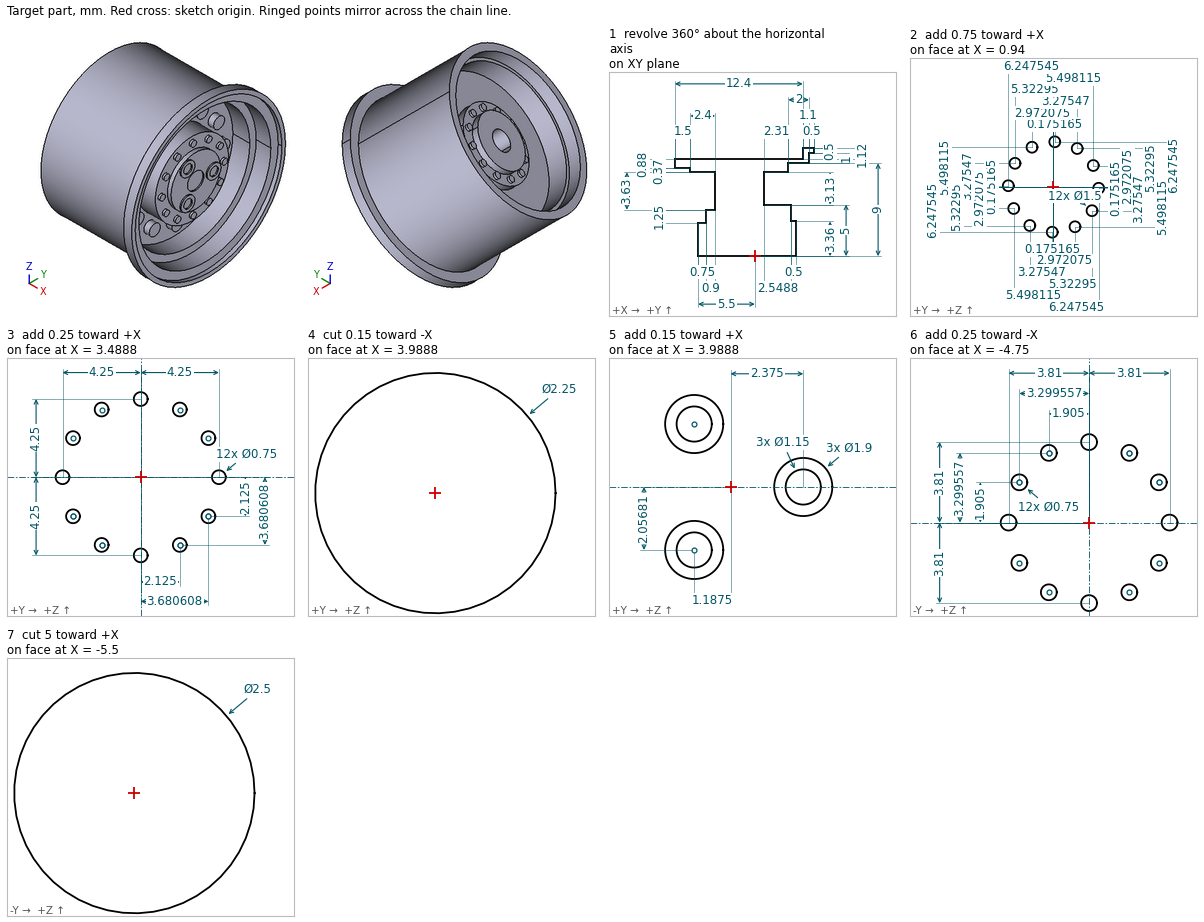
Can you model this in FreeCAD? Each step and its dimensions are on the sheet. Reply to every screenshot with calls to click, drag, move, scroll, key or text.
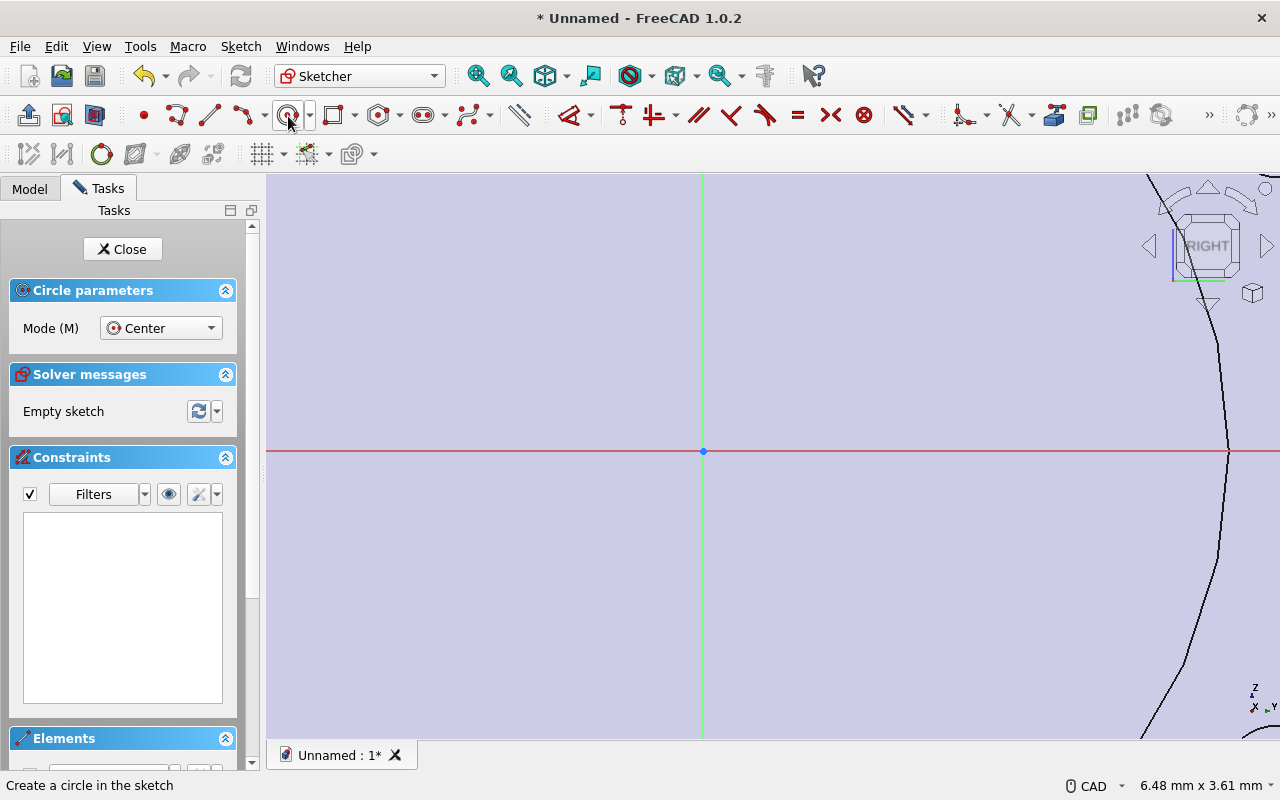
click(703, 451)
move(828, 327)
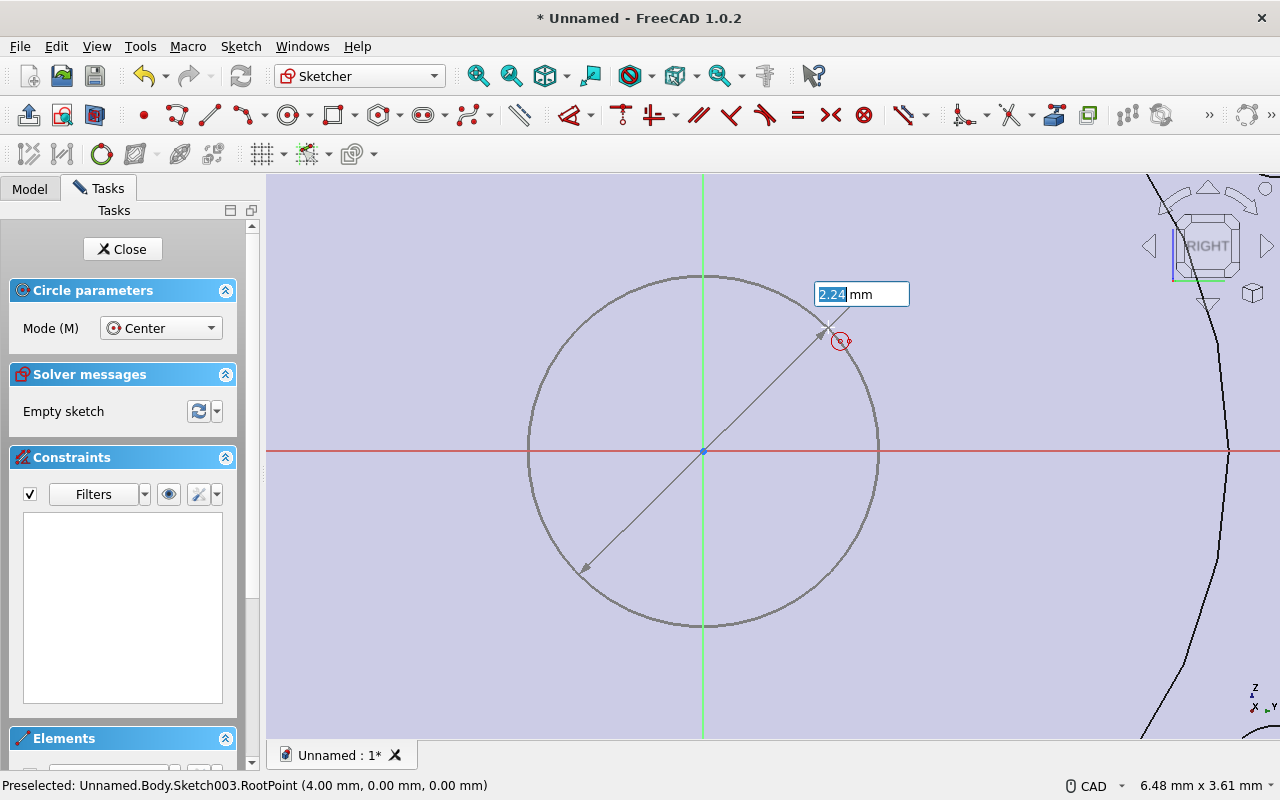
text(2.25)
key(Return)
key(Escape)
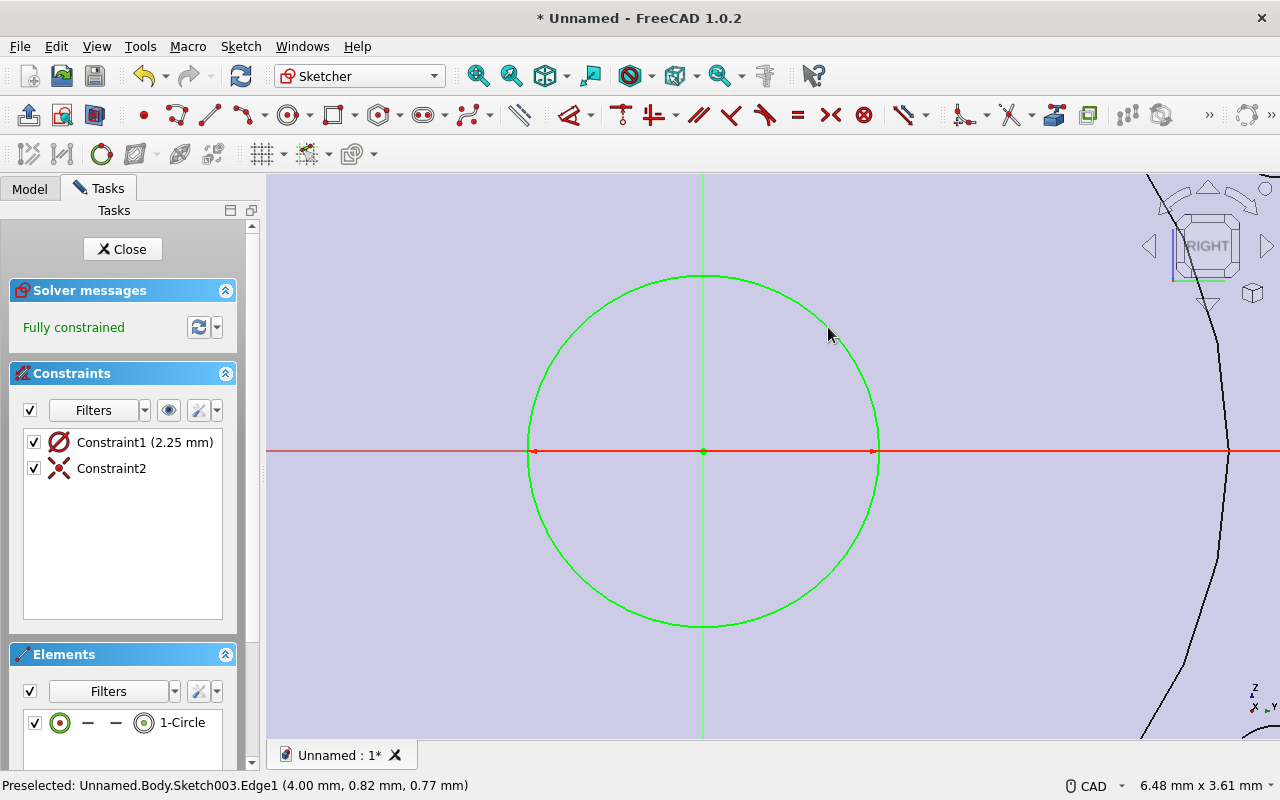
click(123, 249)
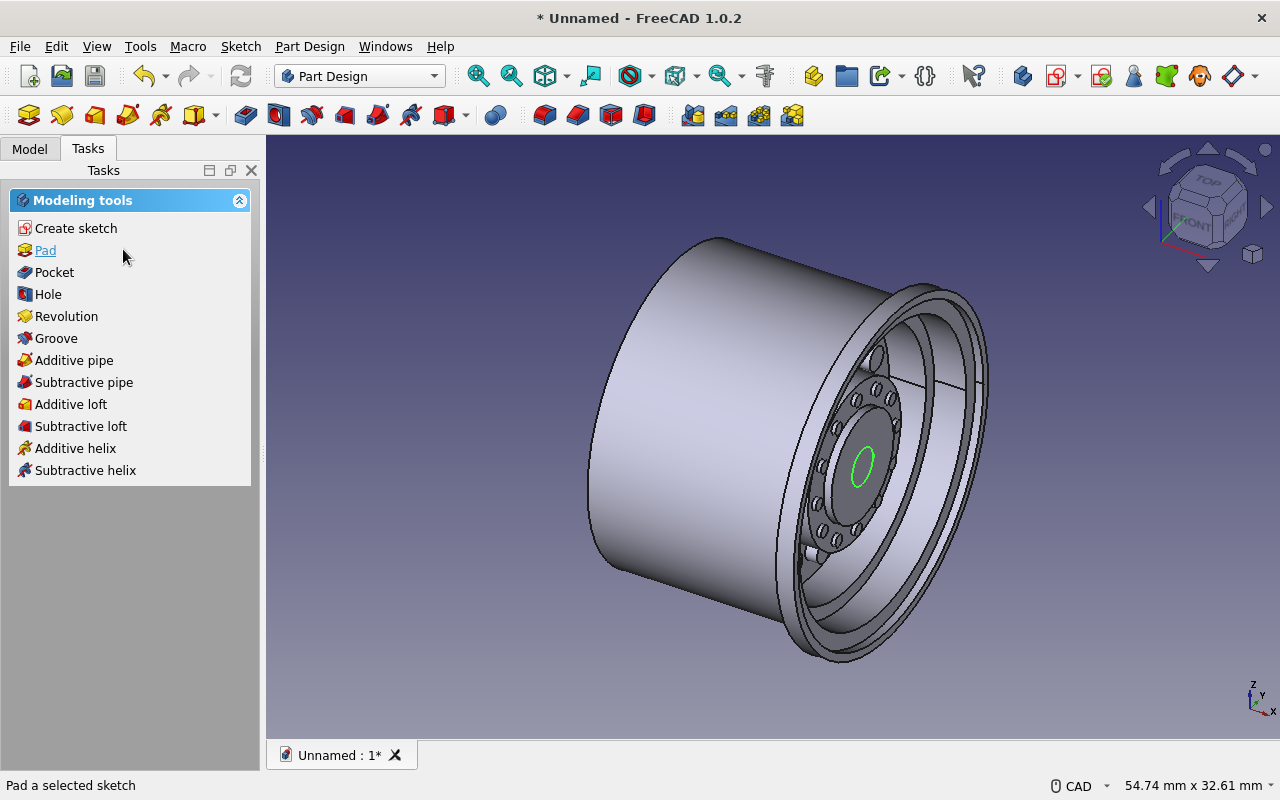
click(246, 116)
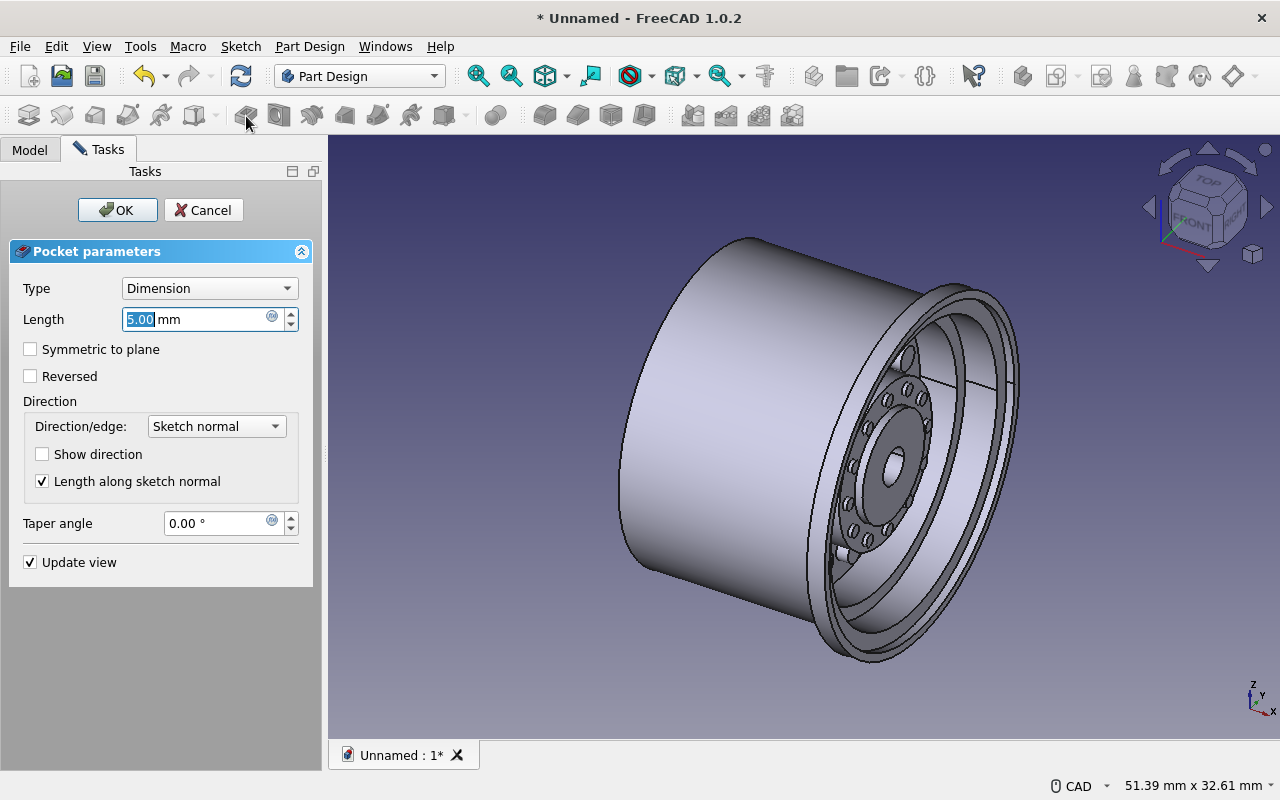
text(0.15)
key(Tab)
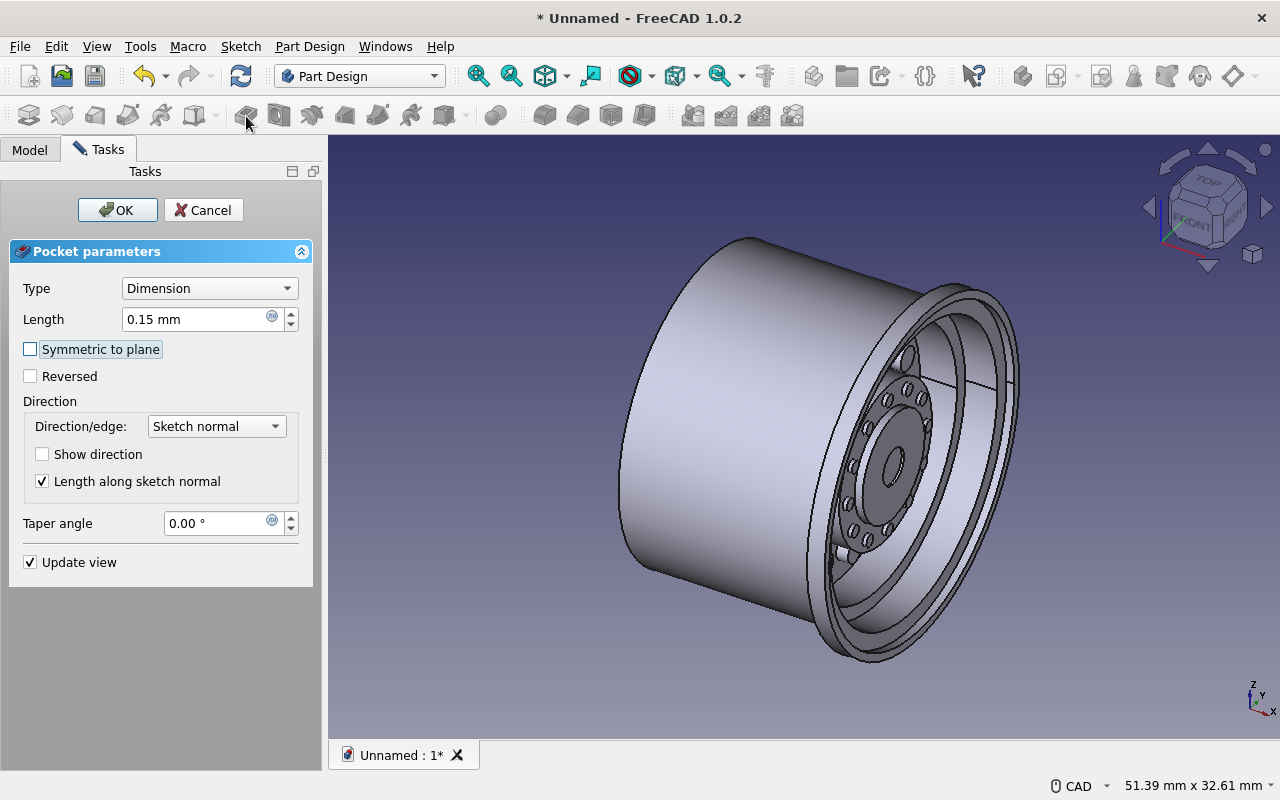
click(118, 210)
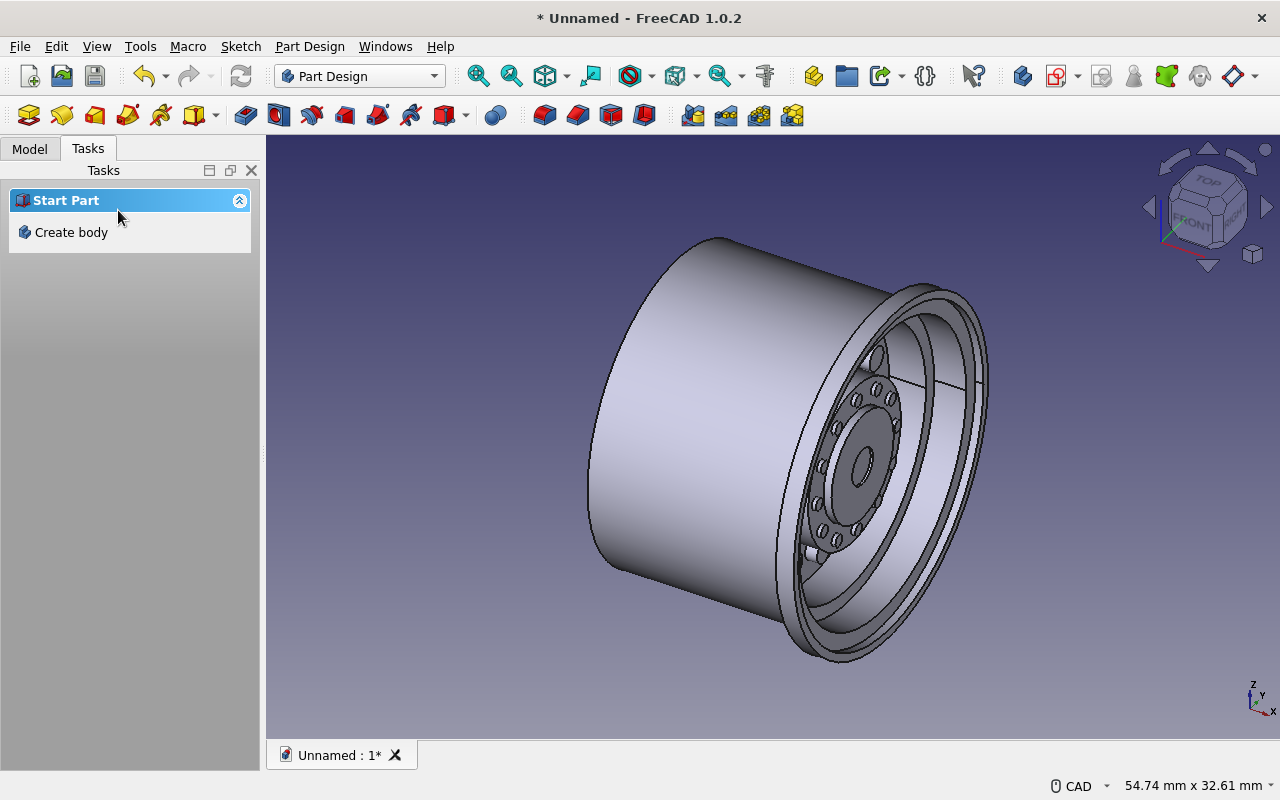
click(872, 428)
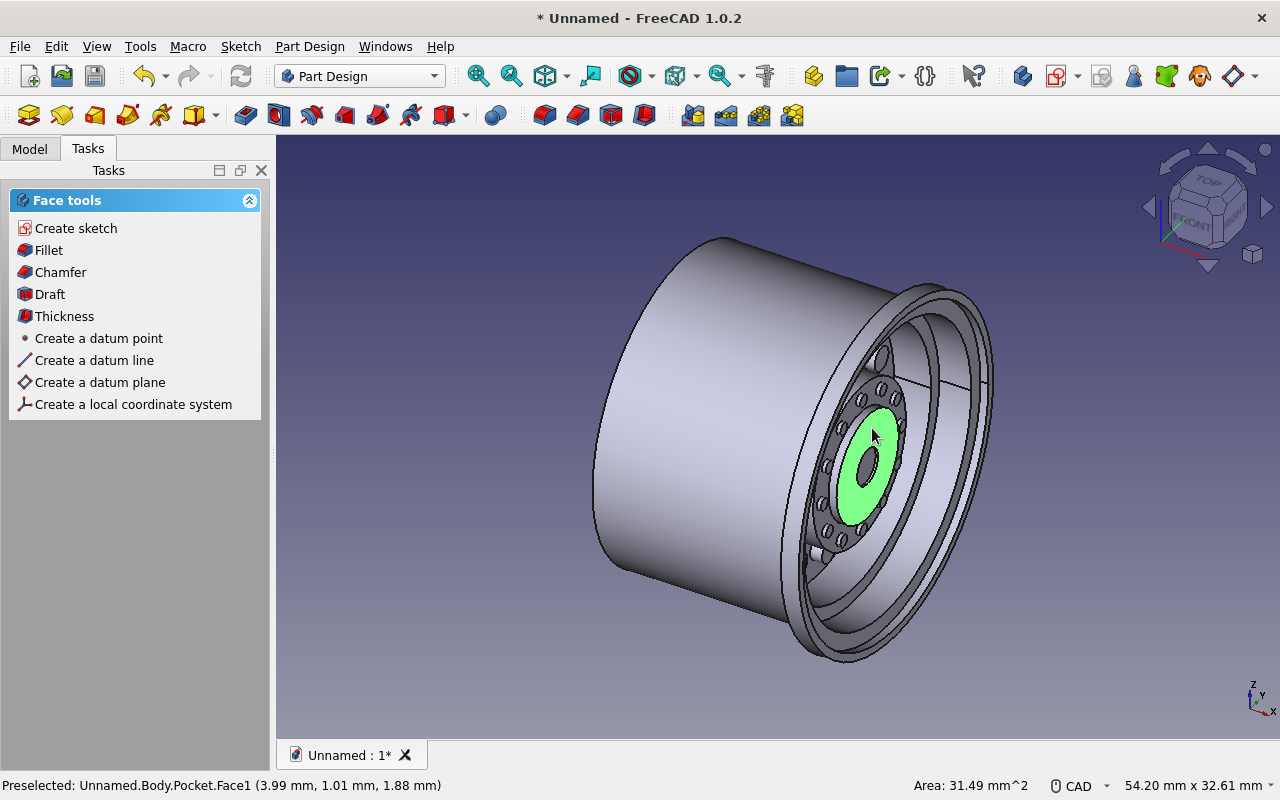
click(1056, 76)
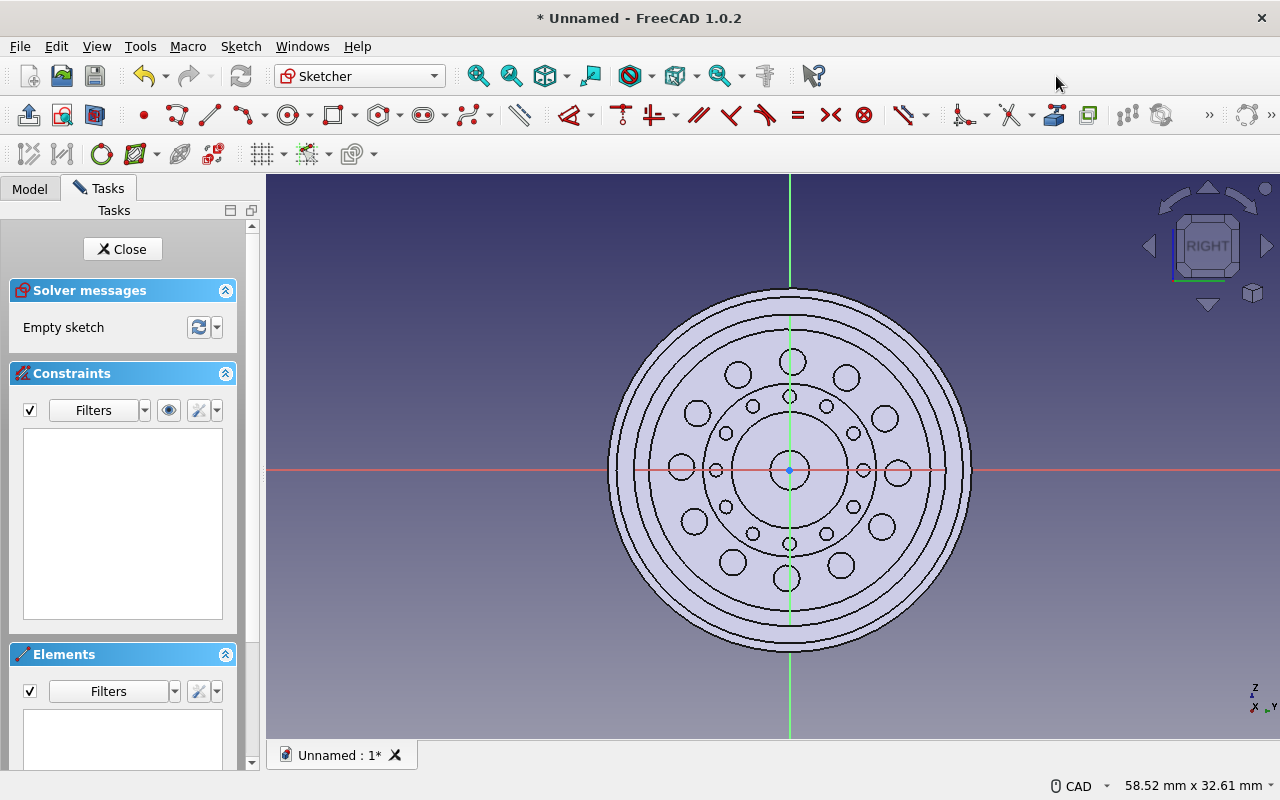
click(95, 116)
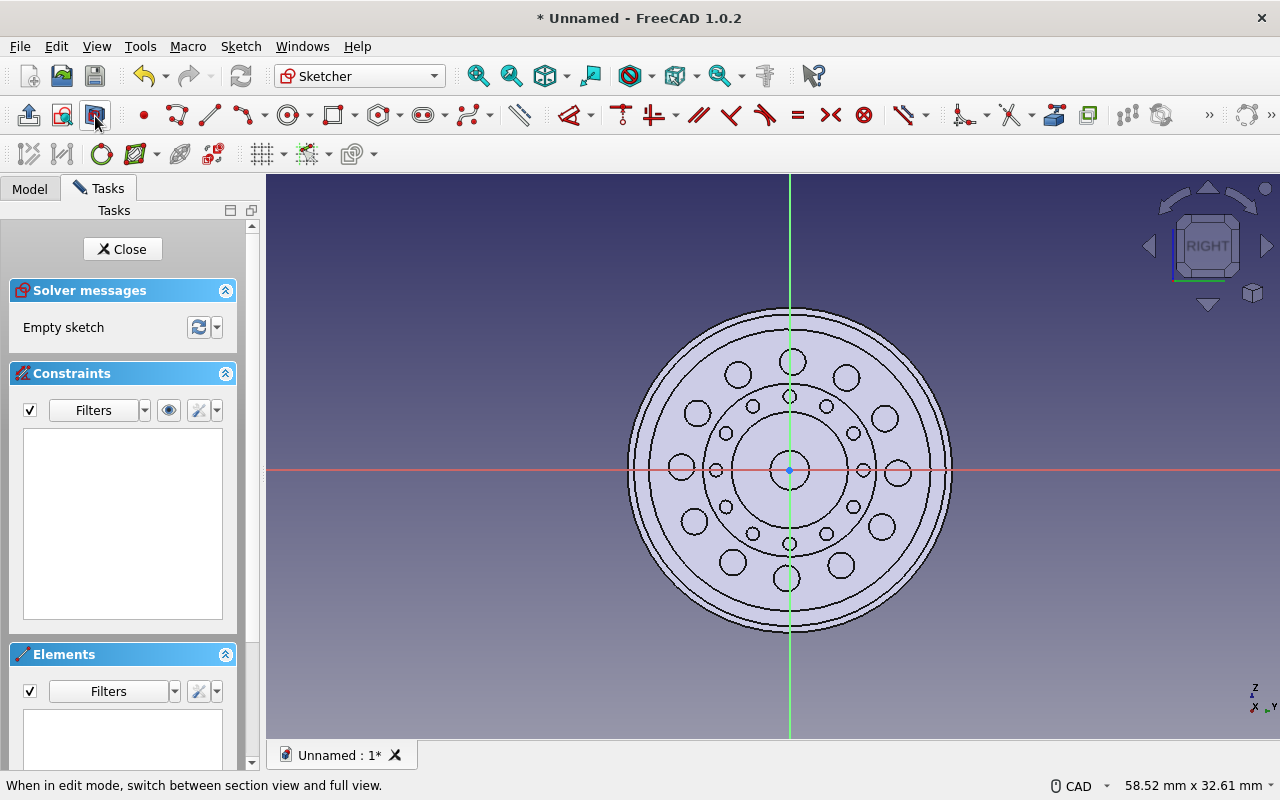
scroll(841, 476, up, 6)